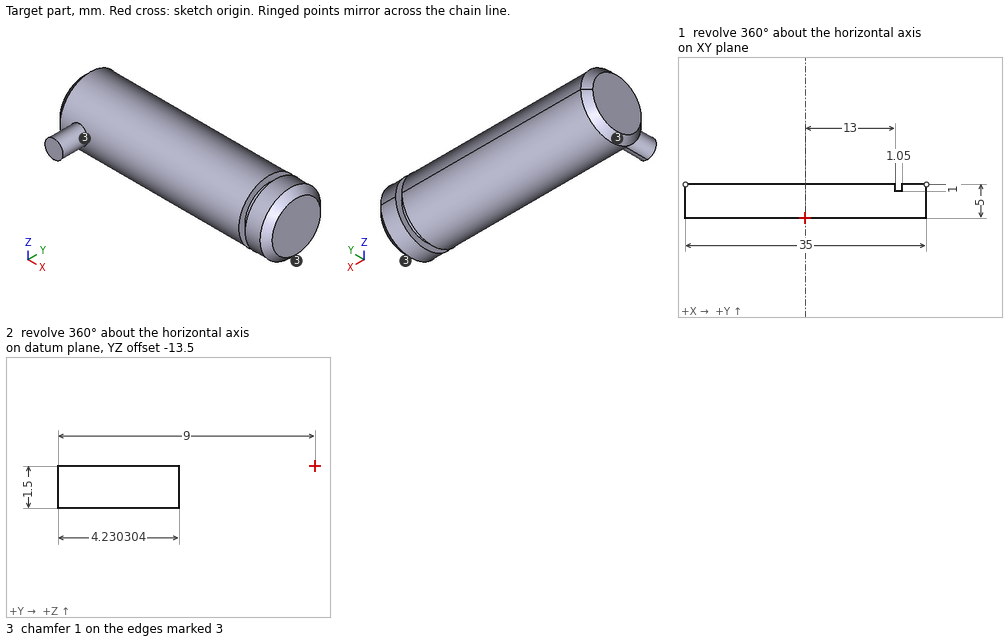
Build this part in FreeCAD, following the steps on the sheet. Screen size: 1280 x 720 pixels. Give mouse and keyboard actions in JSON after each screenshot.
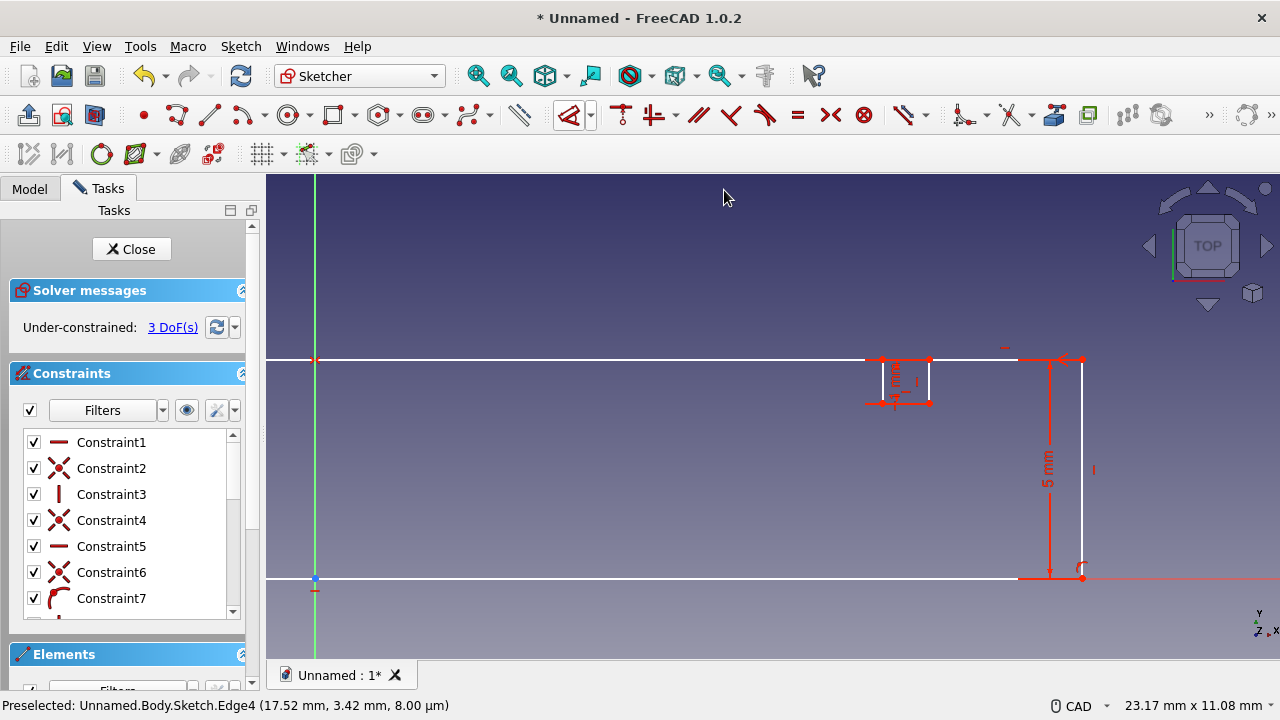
{"action": "left_click", "coordinate": [622, 579]}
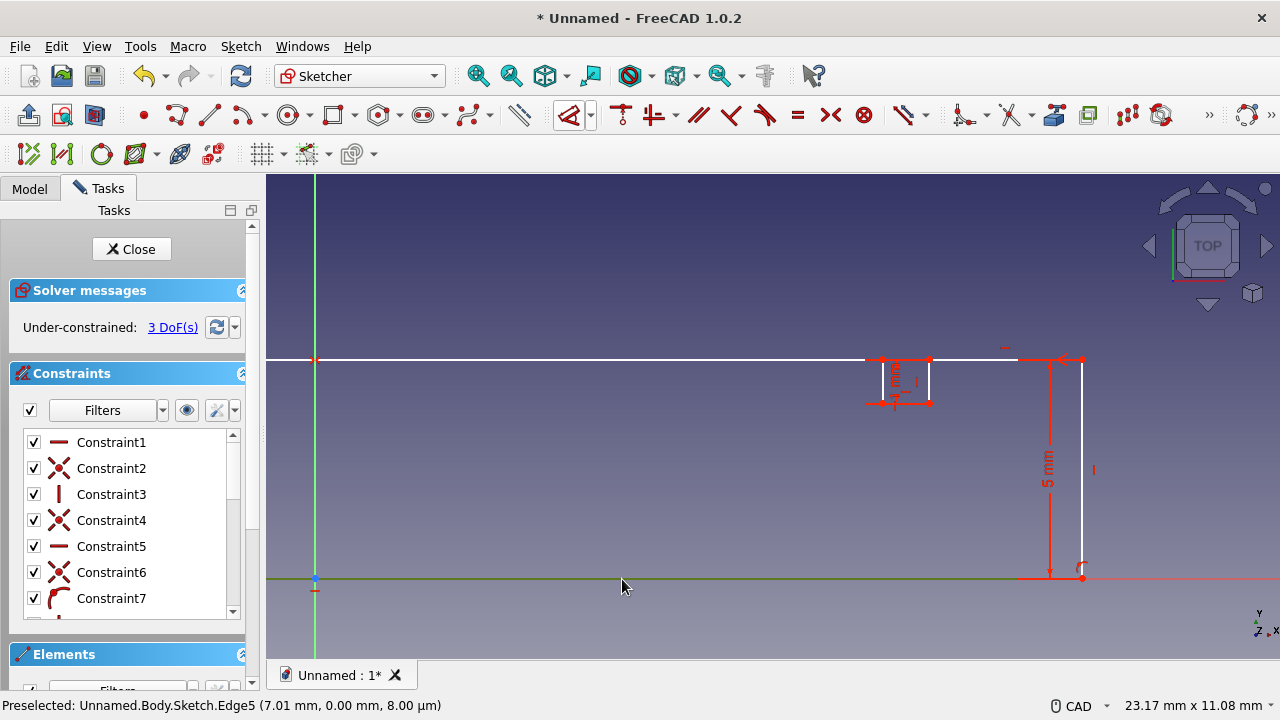
{"action": "left_click", "coordinate": [590, 116]}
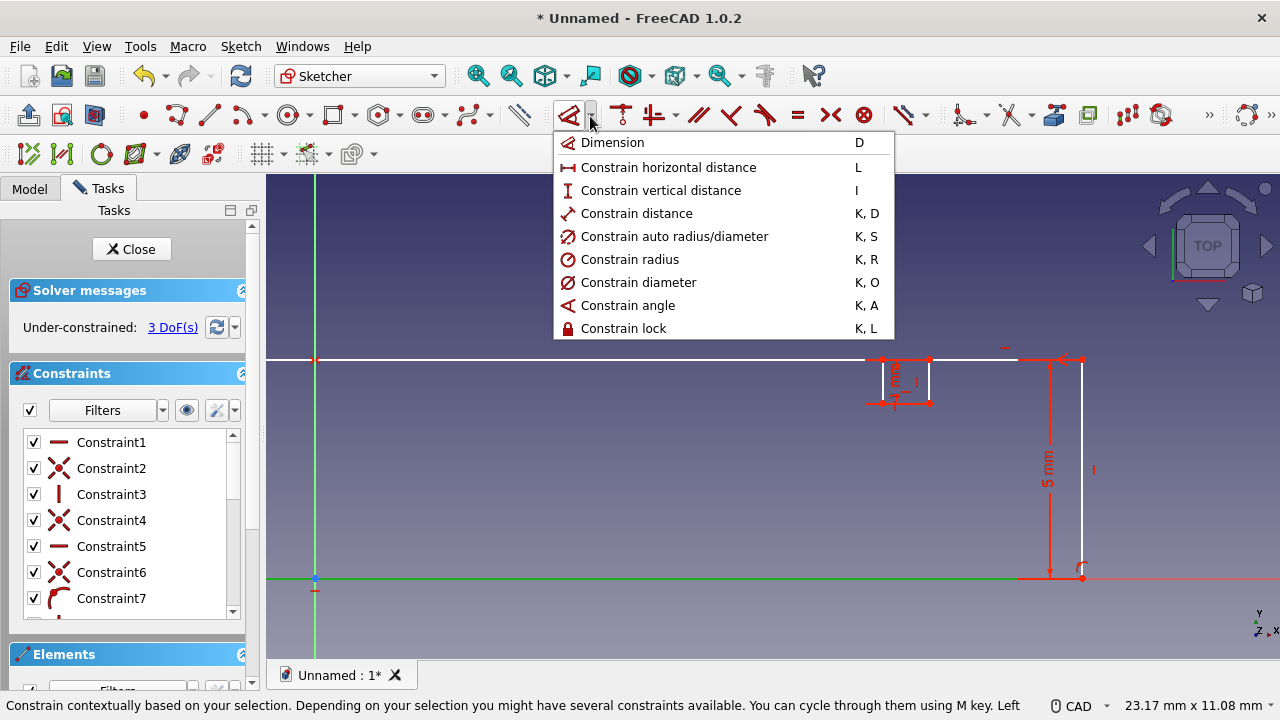
{"action": "left_click", "coordinate": [724, 168]}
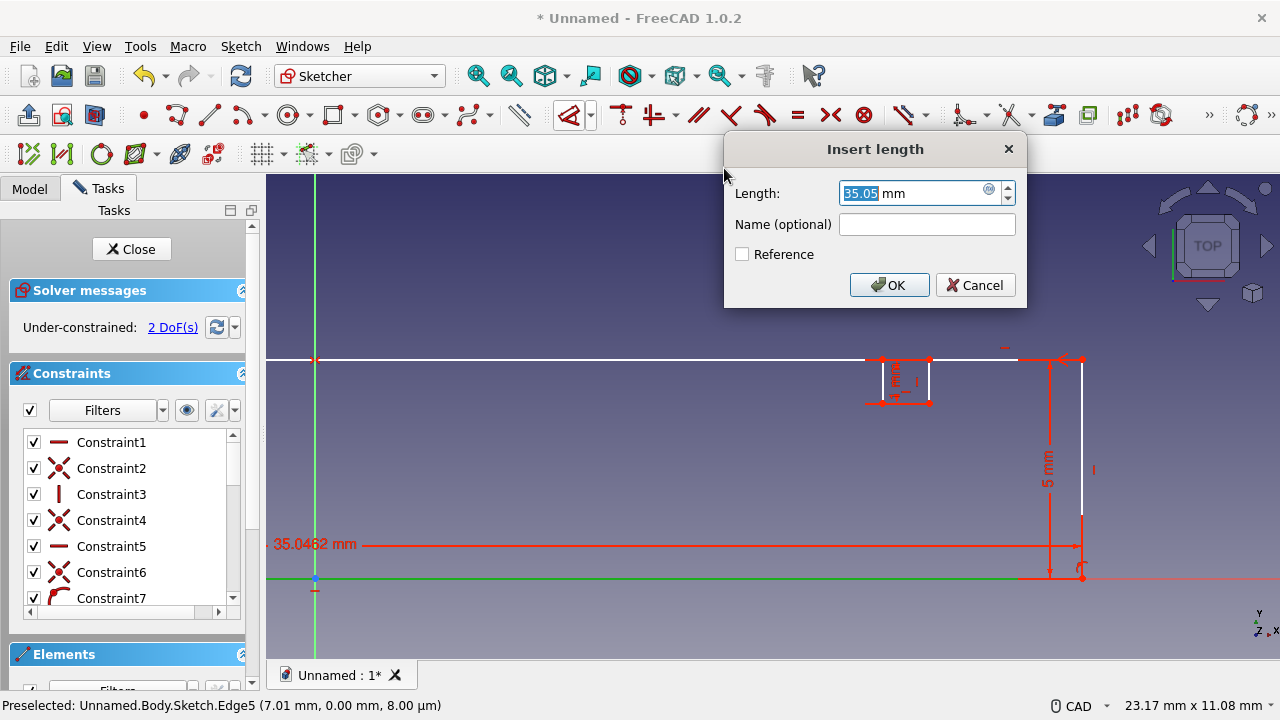
{"action": "type", "text": "35"}
{"action": "key", "text": "Return"}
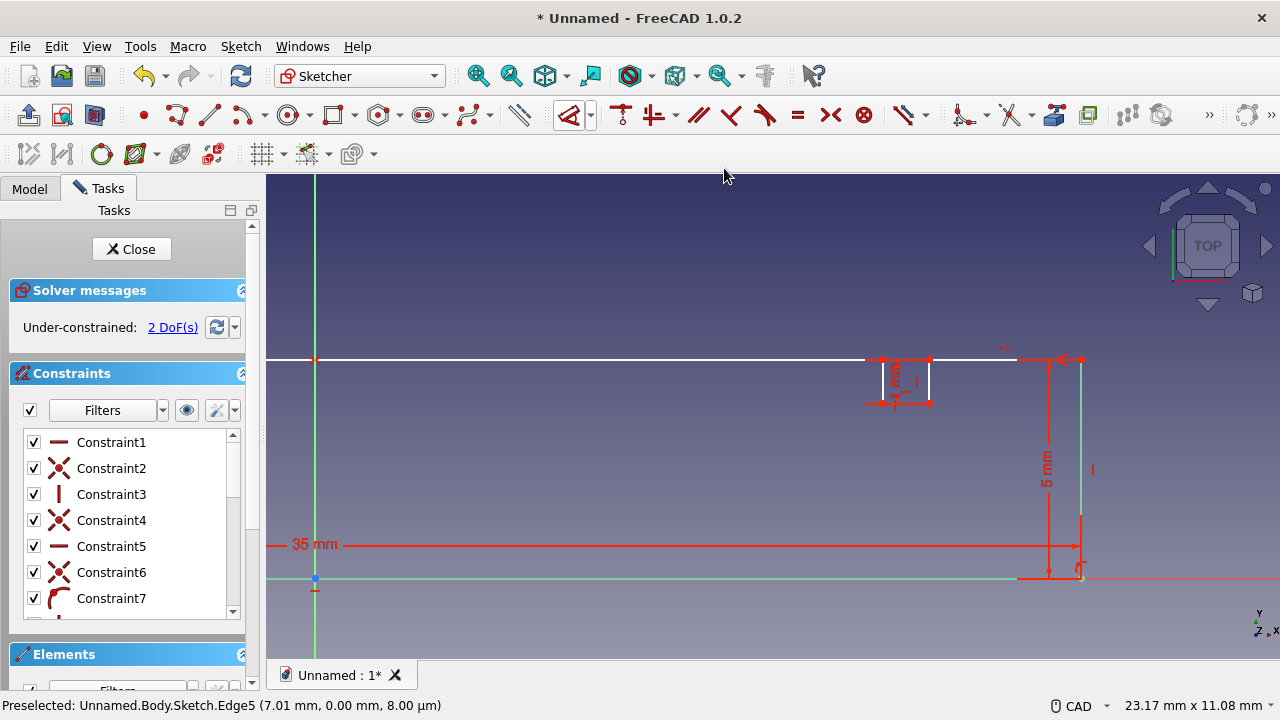
{"action": "left_click", "coordinate": [883, 404]}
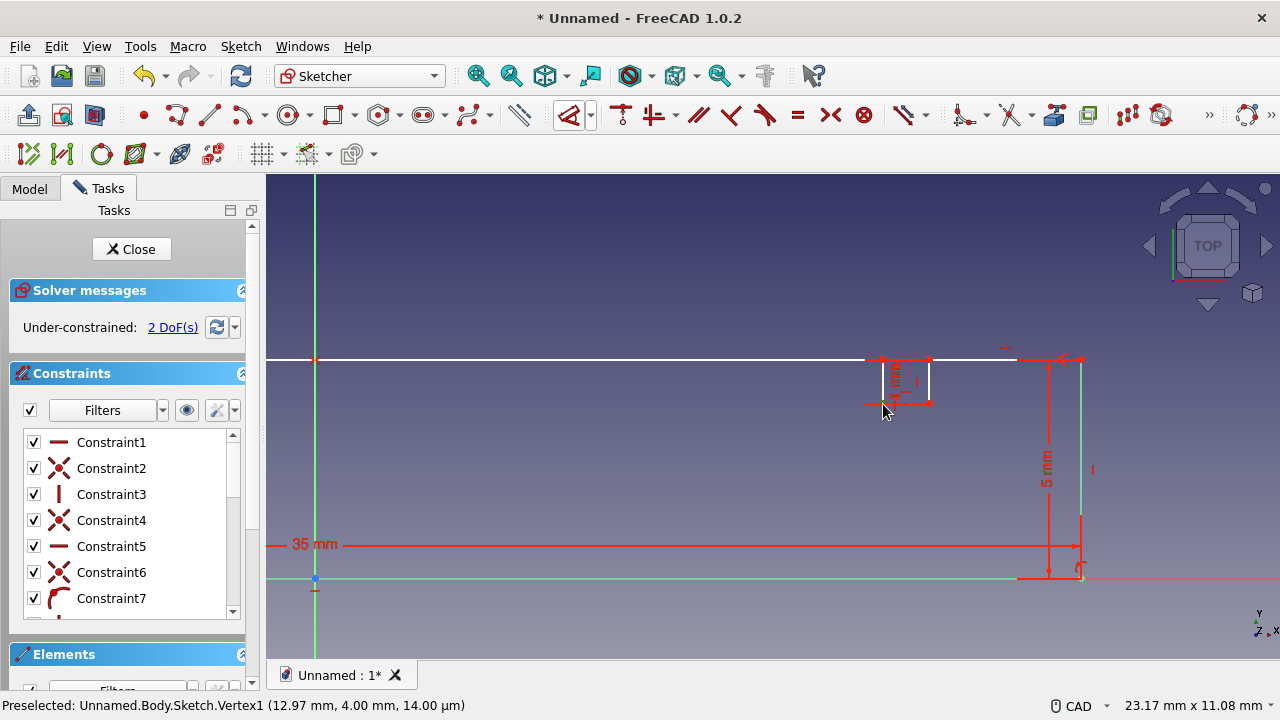
{"action": "key", "text": "l"}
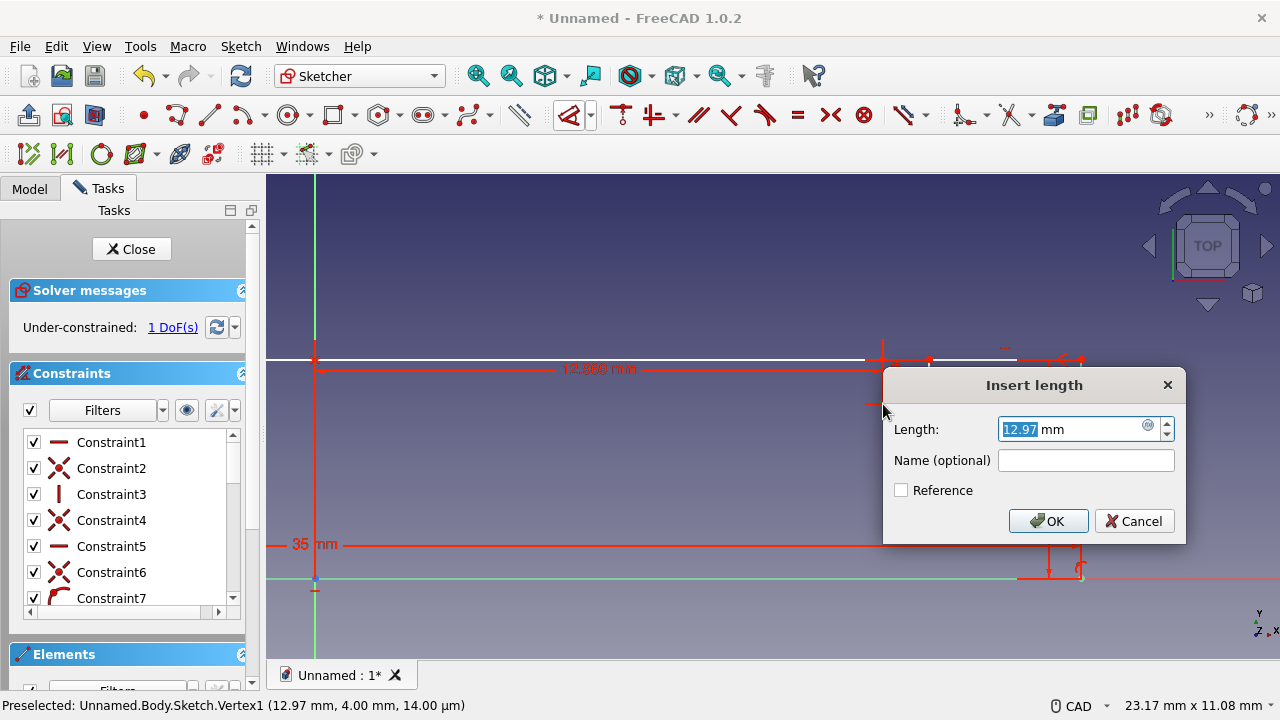
{"action": "type", "text": "13"}
{"action": "key", "text": "Return"}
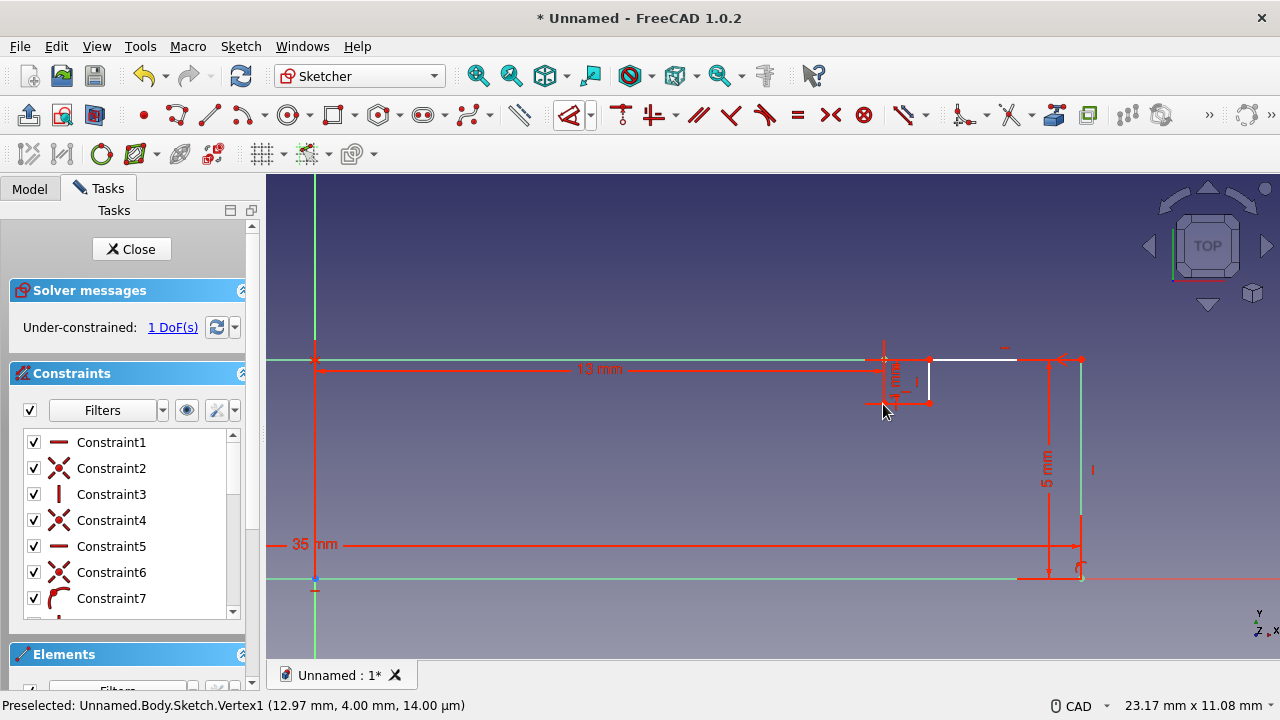
{"action": "left_click", "coordinate": [916, 404]}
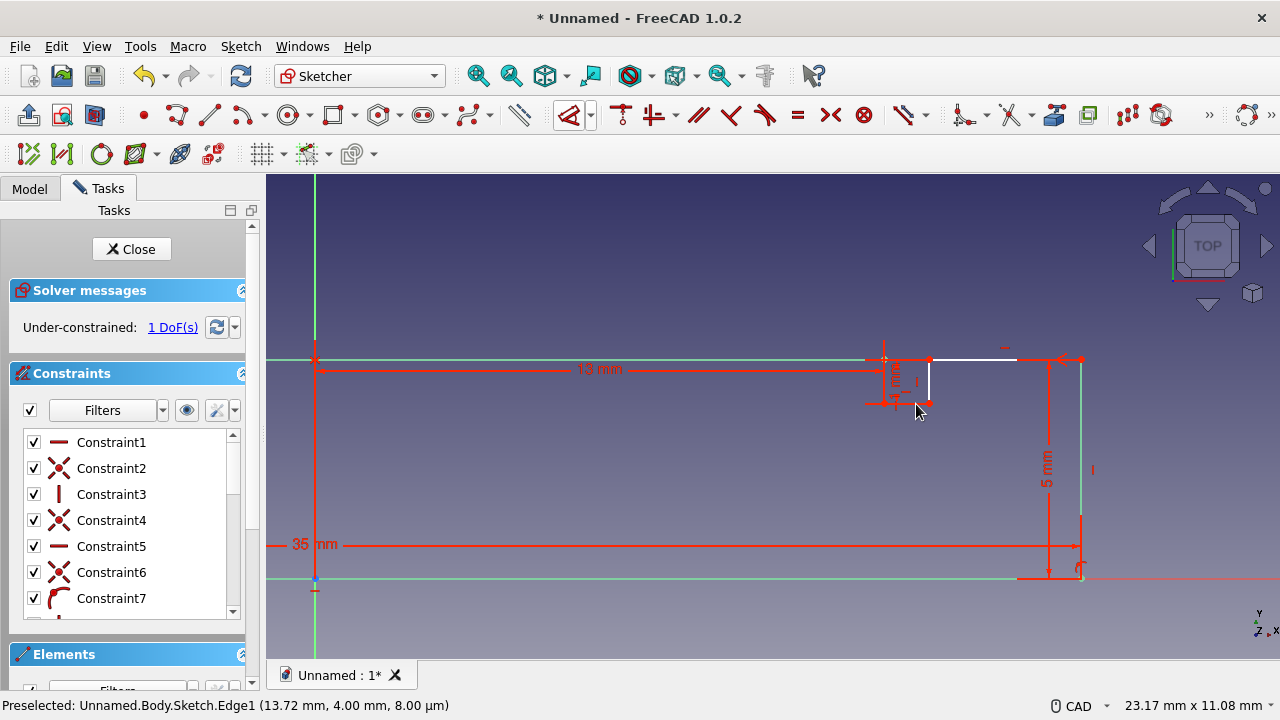
{"action": "key", "text": "l"}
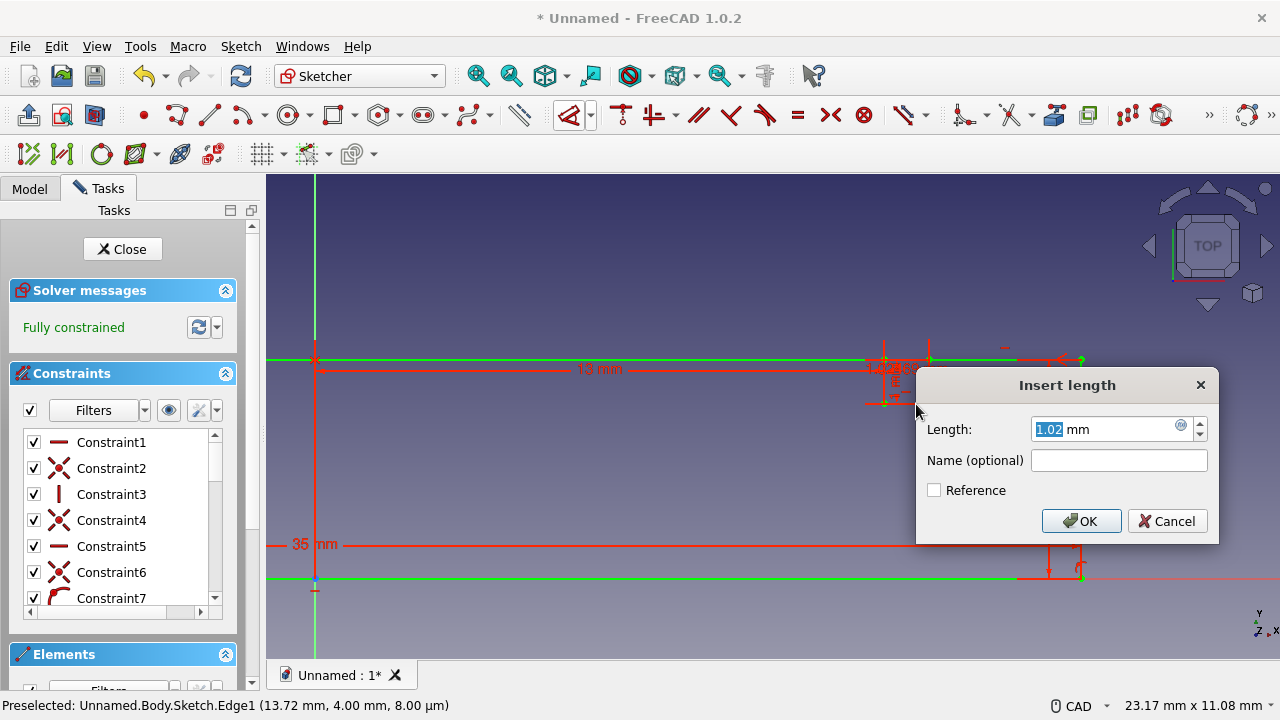
{"action": "type", "text": "1.05"}
{"action": "key", "text": "Return"}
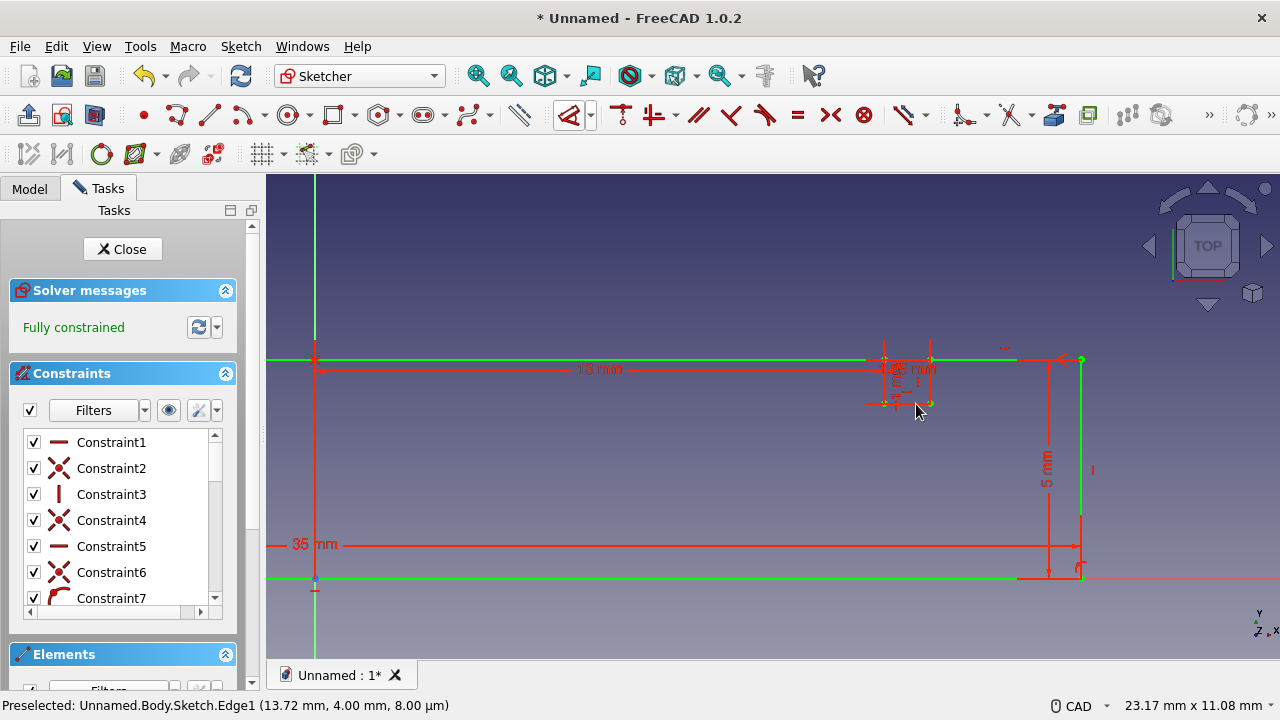
{"action": "left_click", "coordinate": [123, 249]}